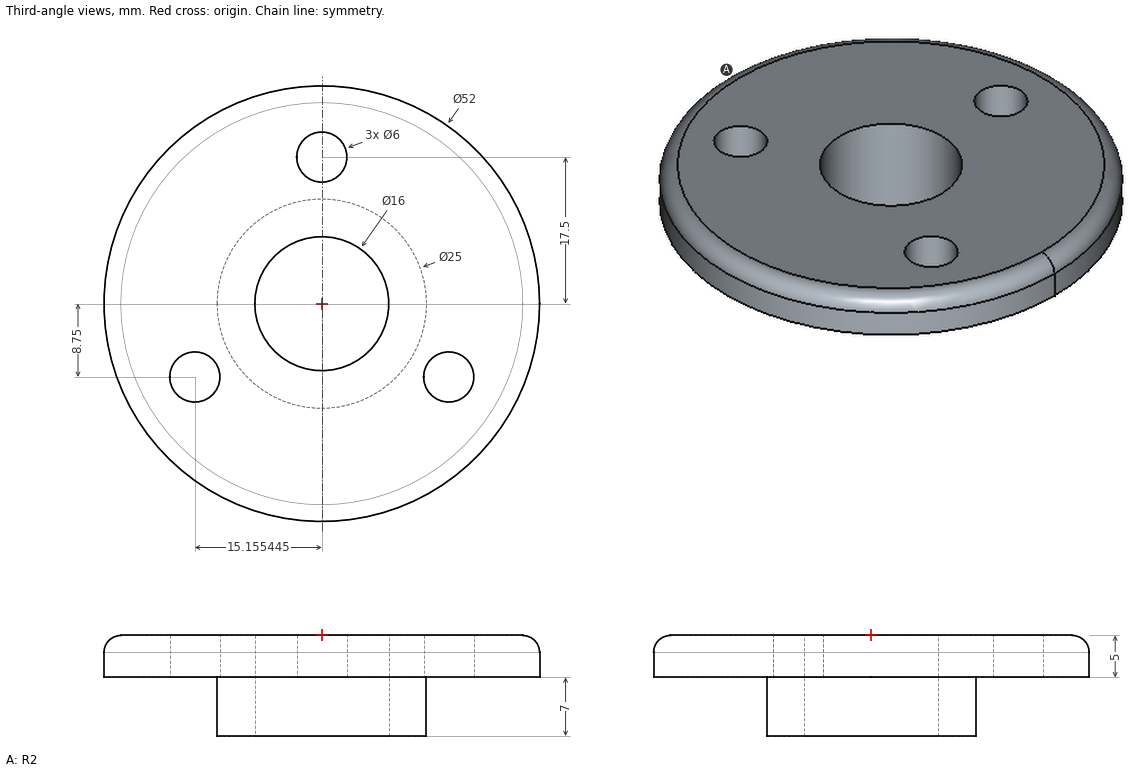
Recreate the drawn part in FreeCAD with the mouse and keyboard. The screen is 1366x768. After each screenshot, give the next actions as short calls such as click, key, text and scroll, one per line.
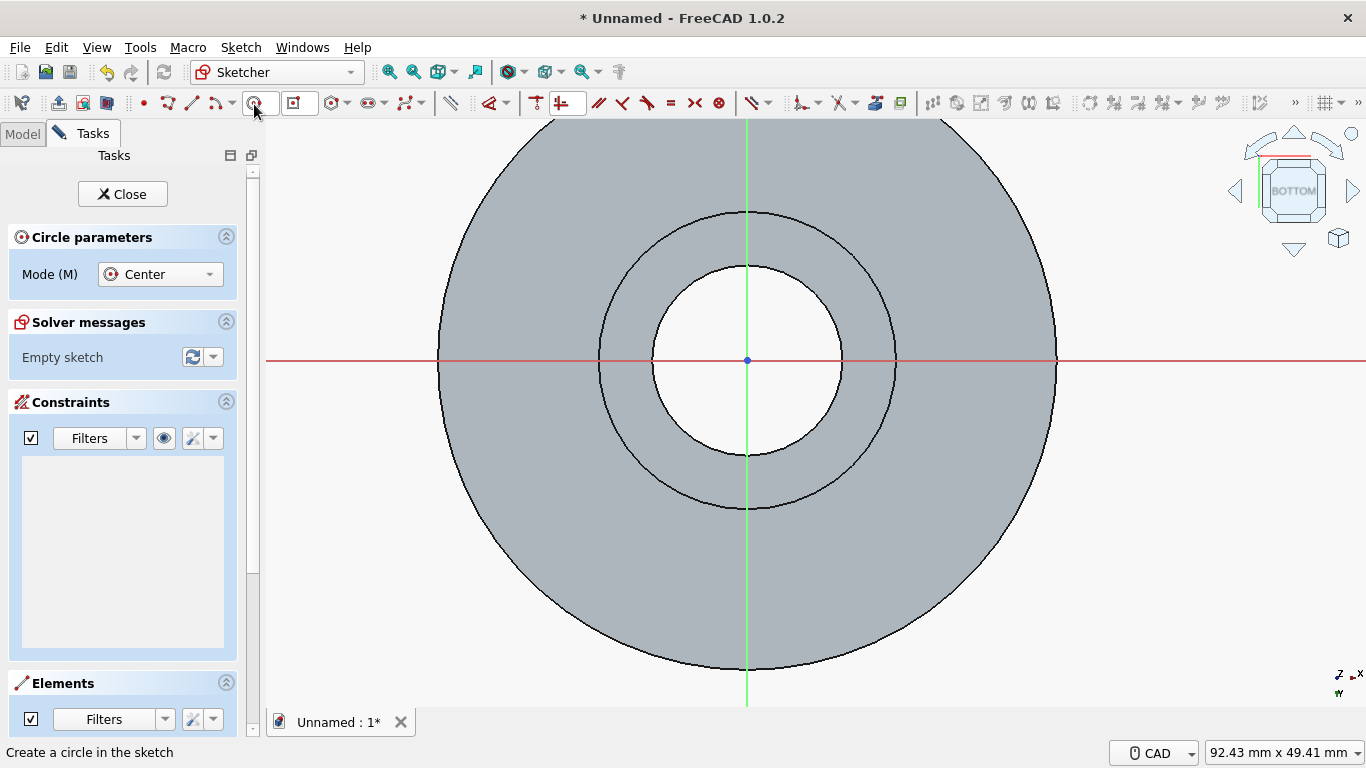
click(747, 569)
move(773, 544)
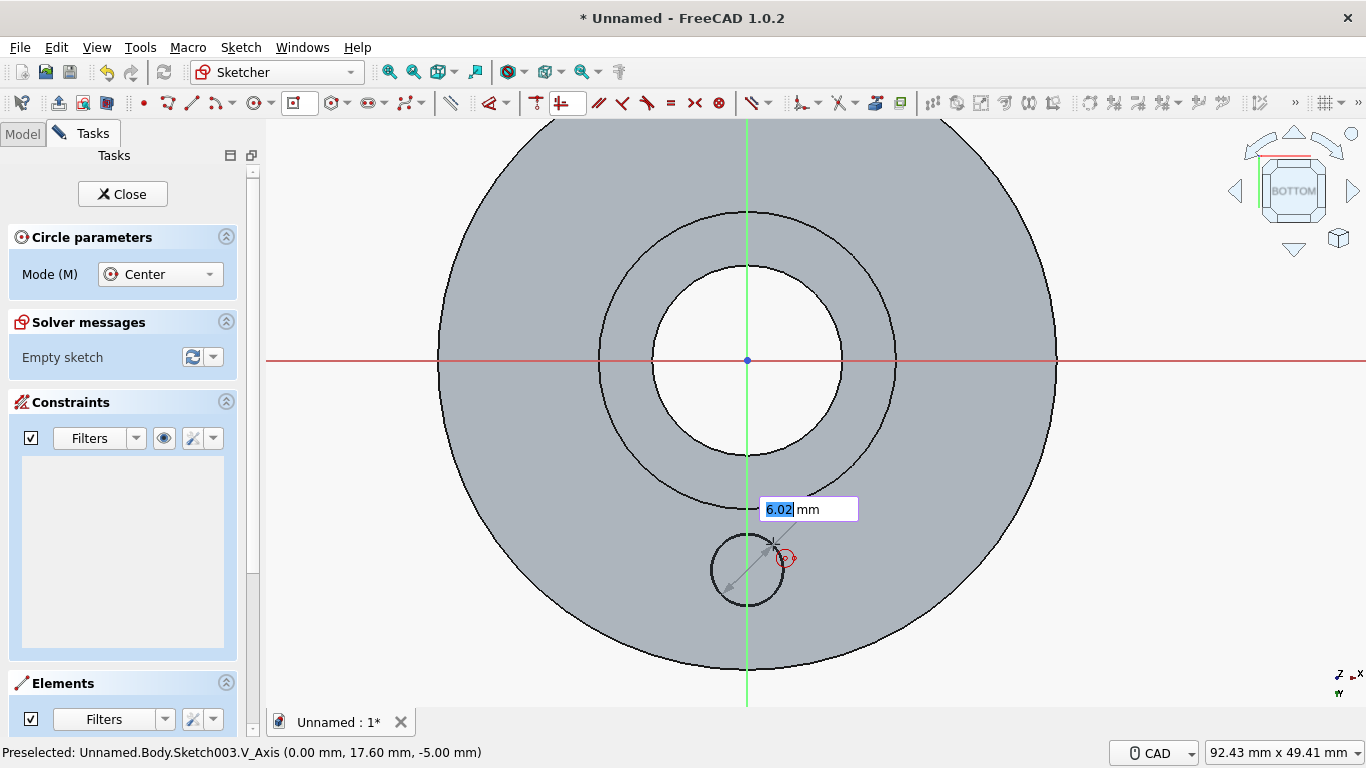
text(6)
key(Return)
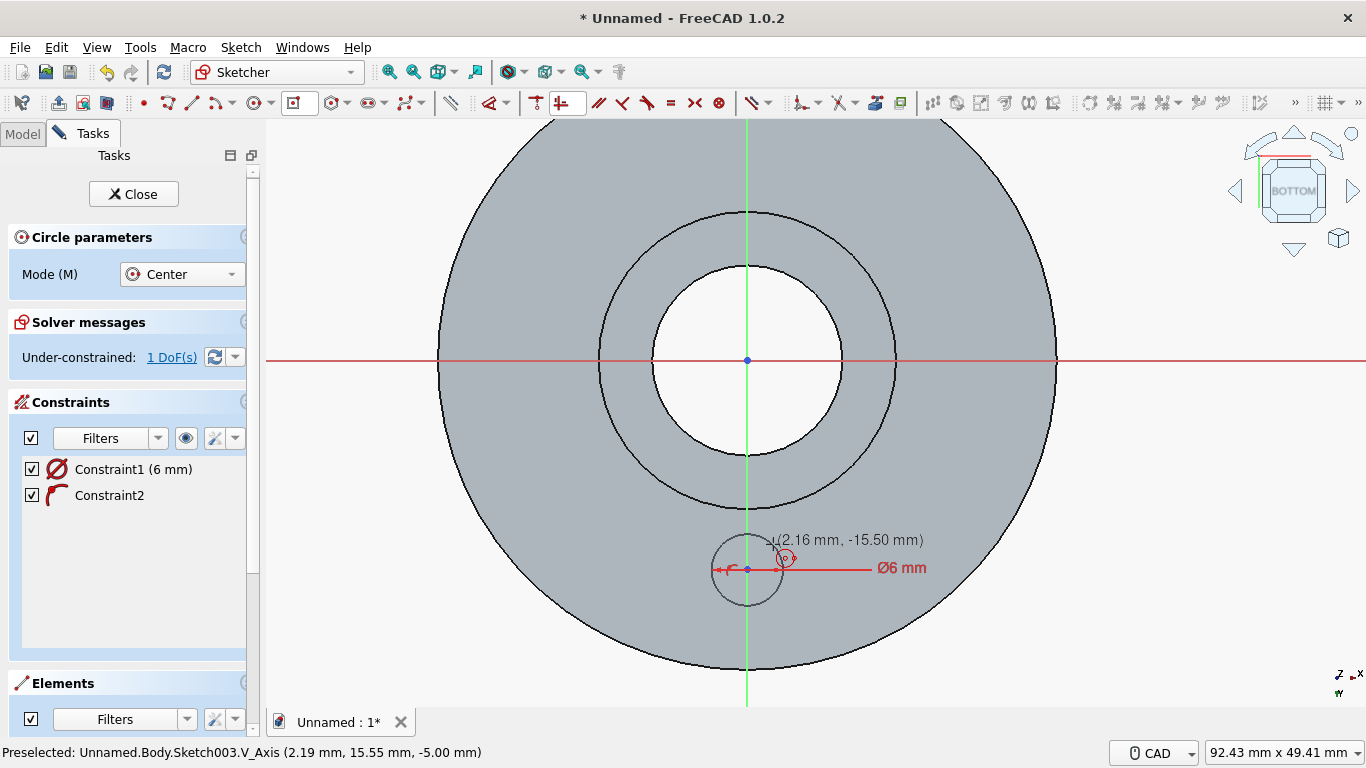
click(567, 256)
move(592, 231)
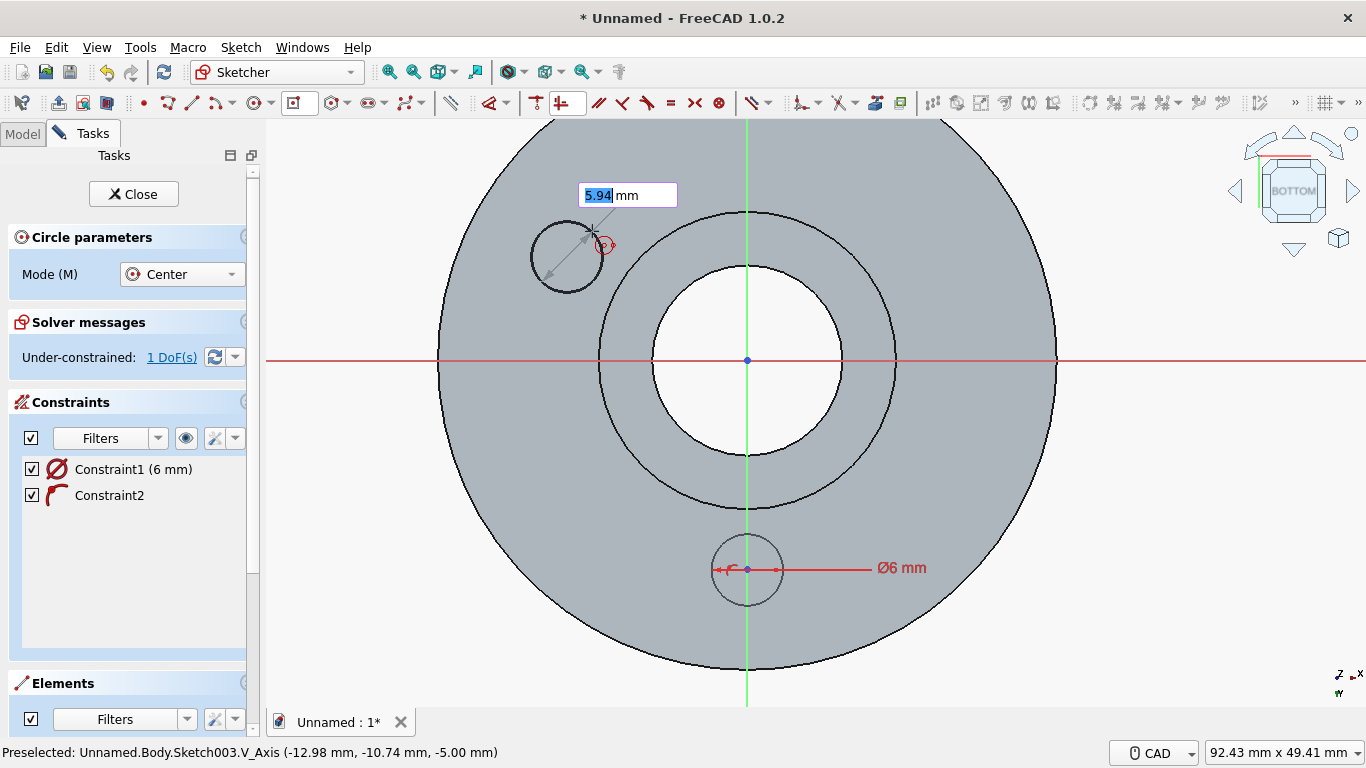
text(6)
key(Return)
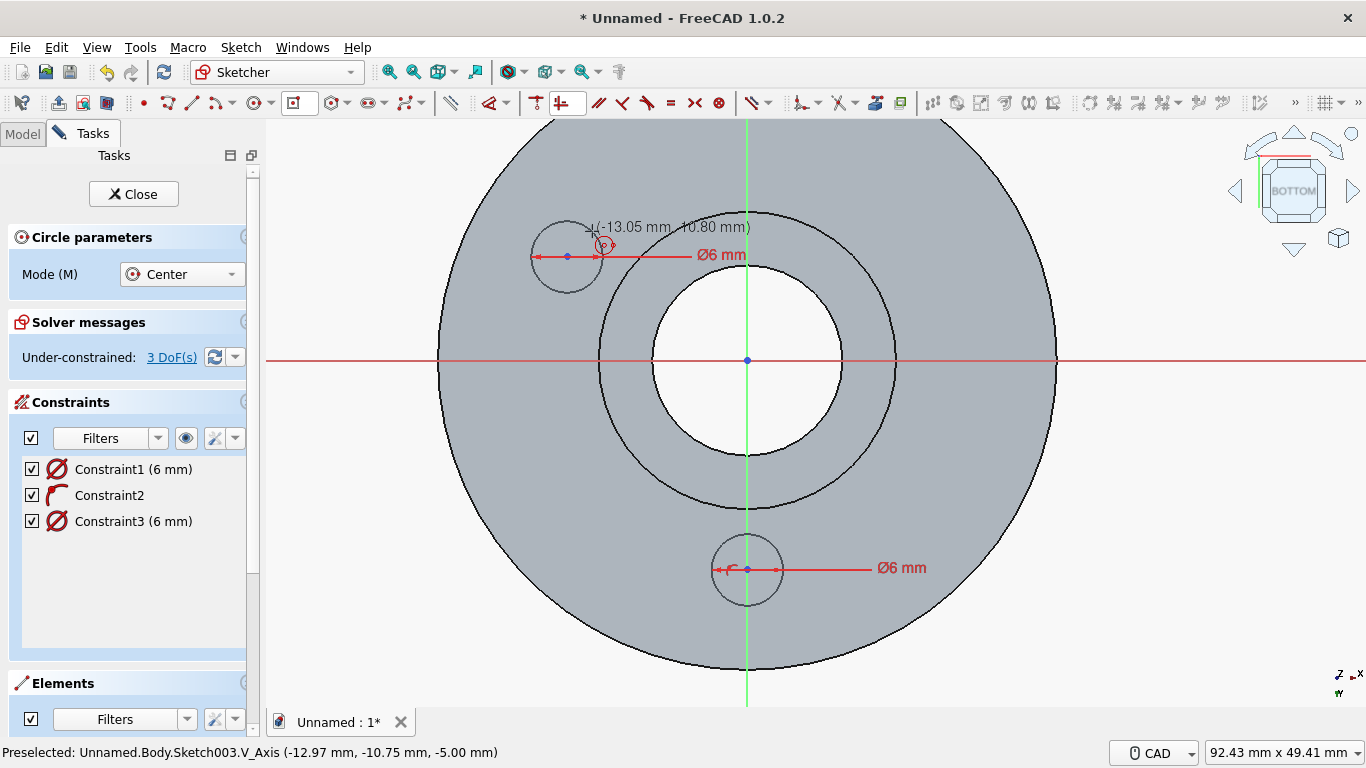
click(928, 256)
move(953, 231)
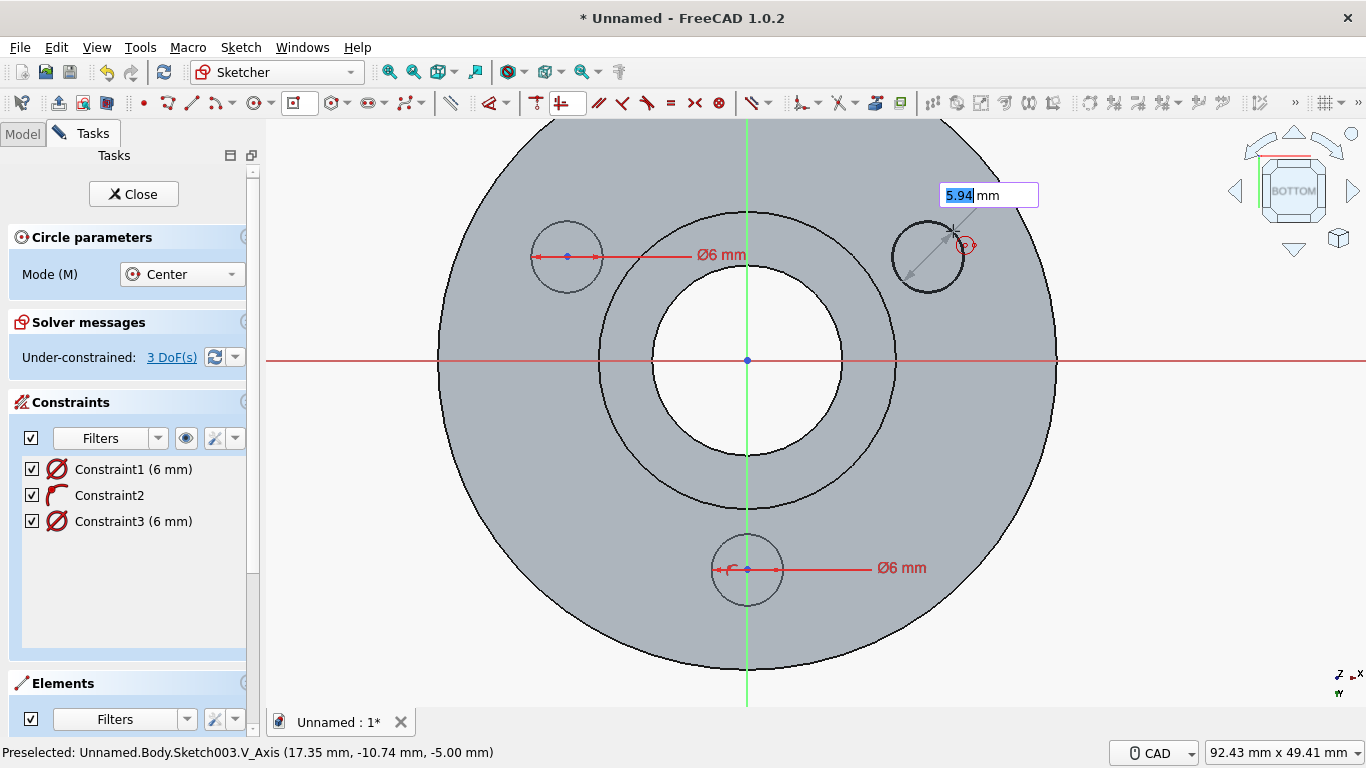
text(6)
key(Return)
key(Escape)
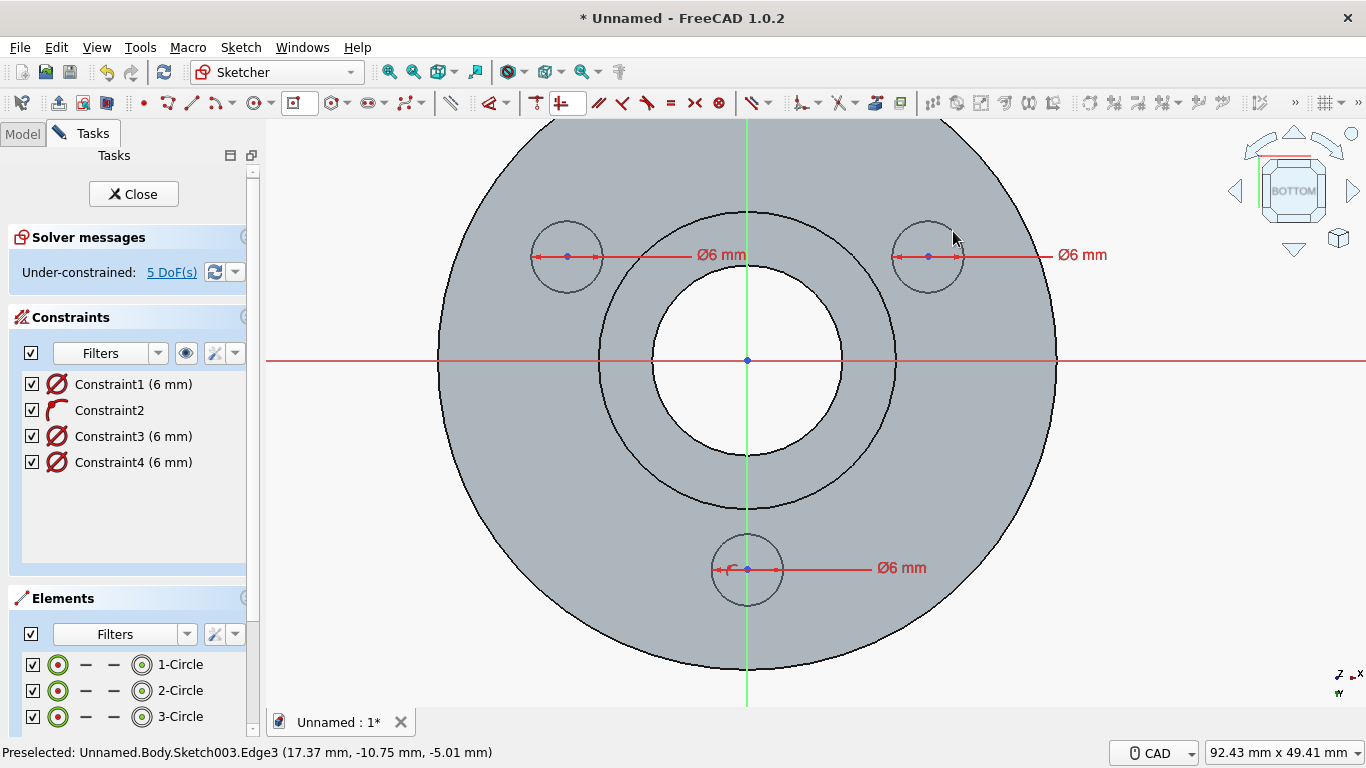
click(567, 257)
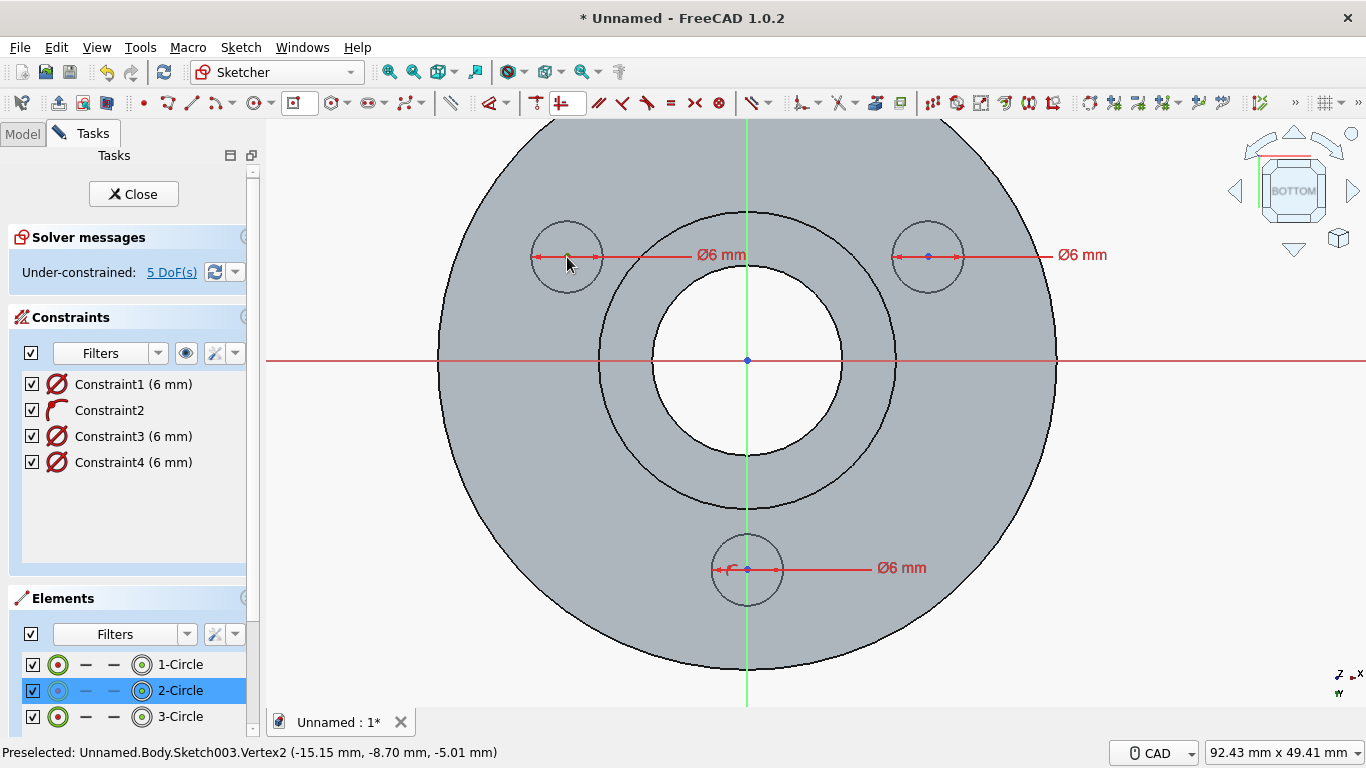
click(928, 257)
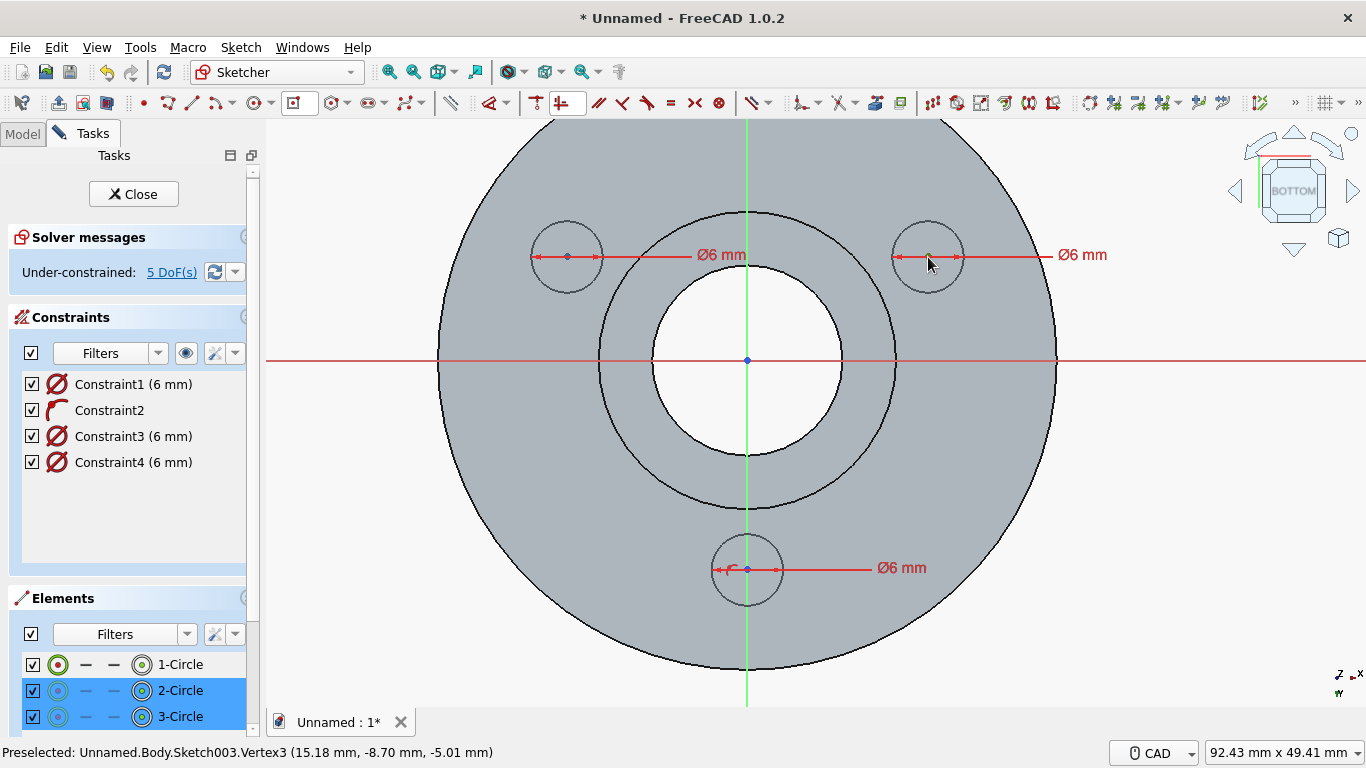
click(747, 641)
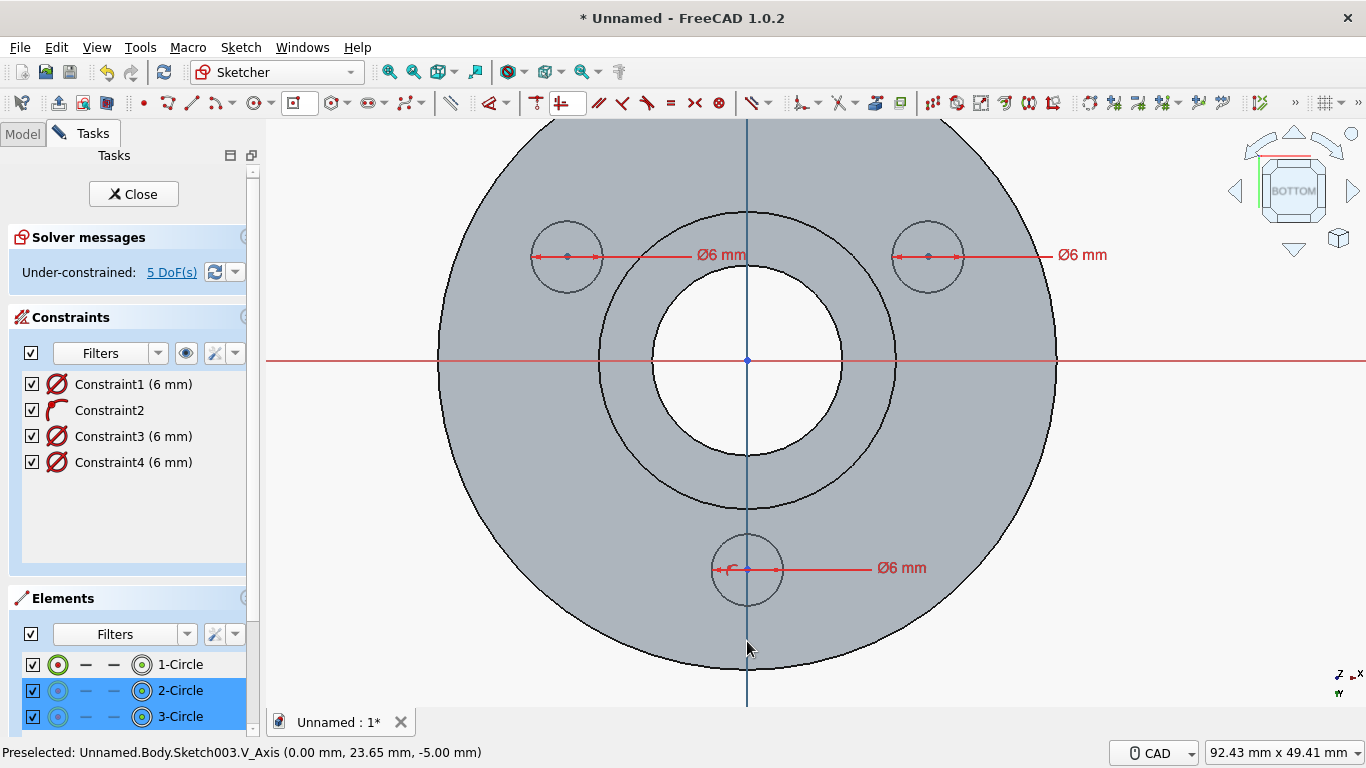
click(696, 104)